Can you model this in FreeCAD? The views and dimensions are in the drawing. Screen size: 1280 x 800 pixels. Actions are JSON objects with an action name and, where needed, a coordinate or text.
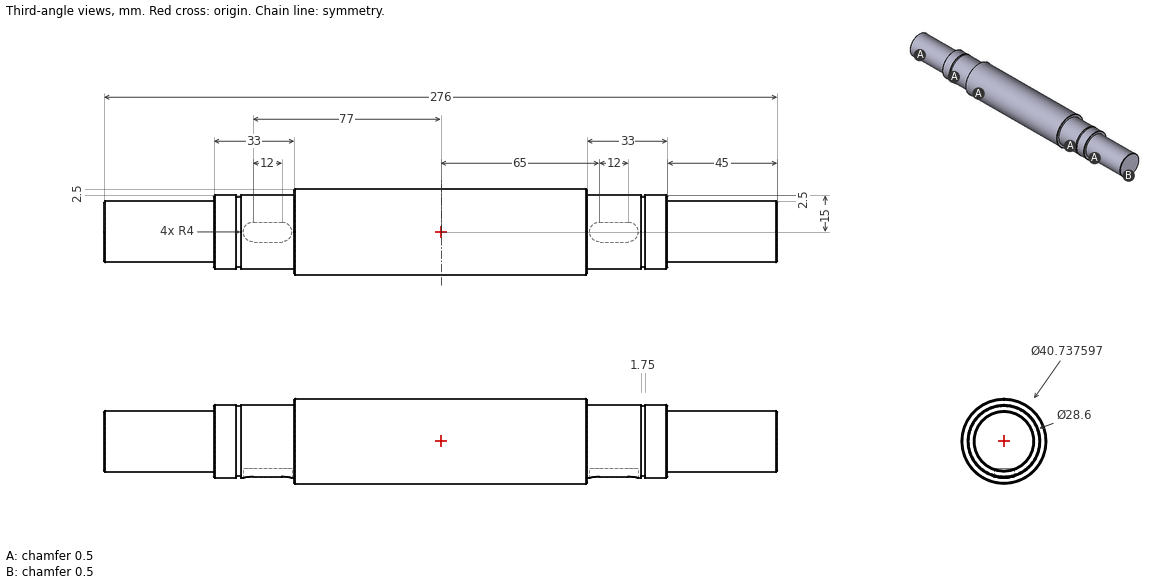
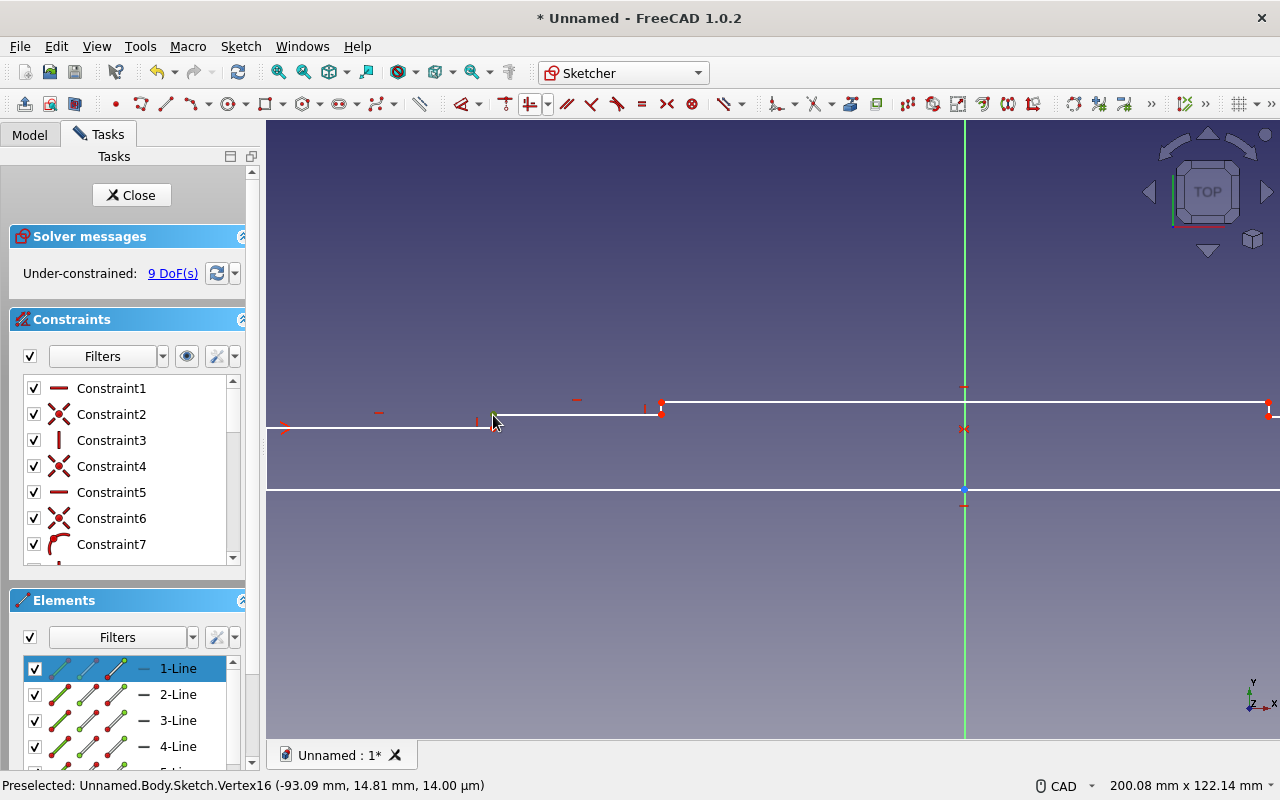
{"action": "left_click", "coordinate": [965, 671]}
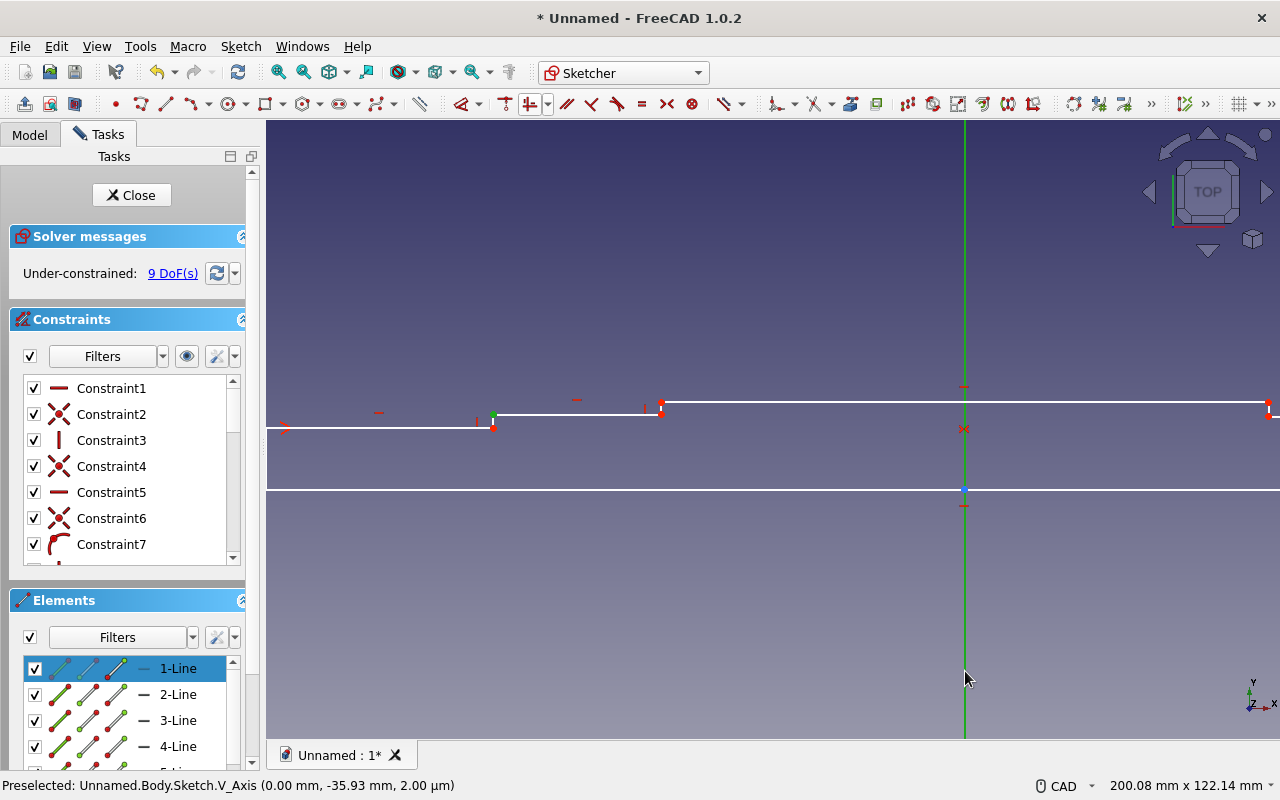
{"action": "left_click", "coordinate": [667, 104]}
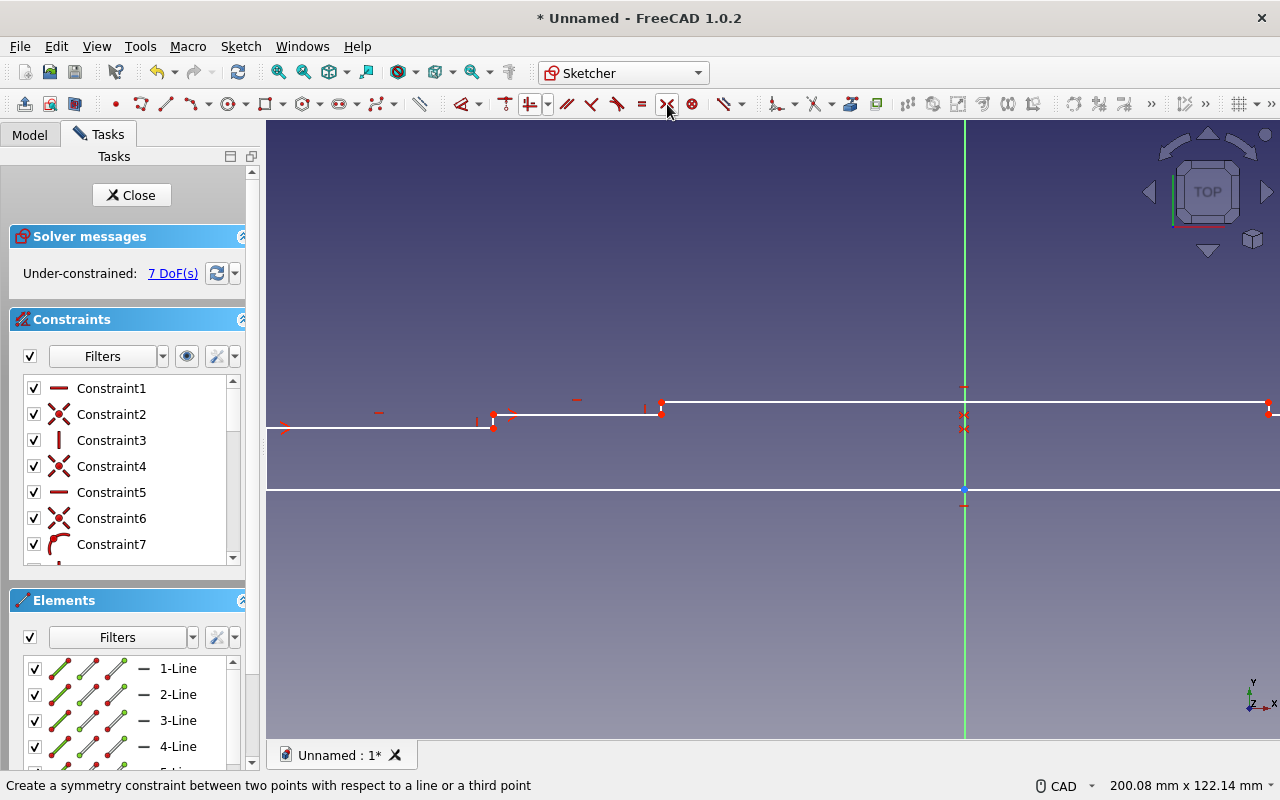
{"action": "left_click", "coordinate": [460, 104]}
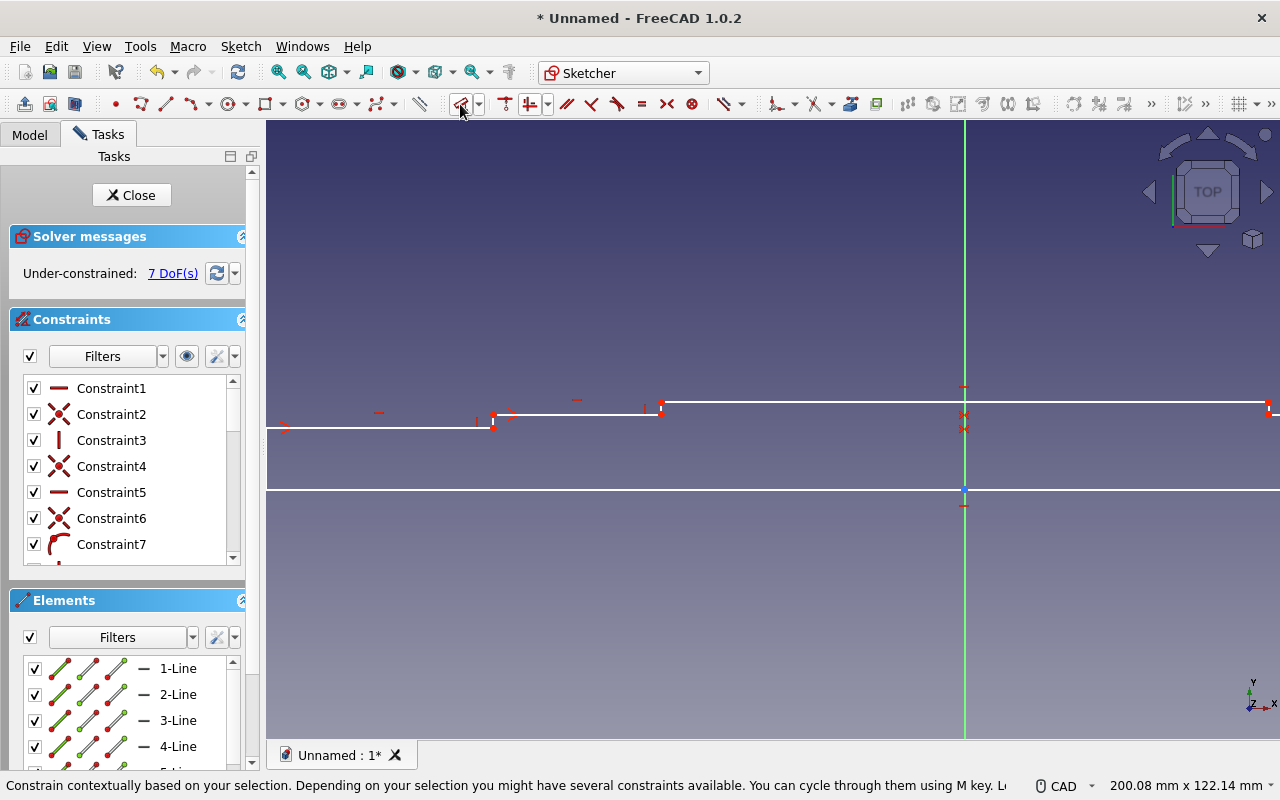
{"action": "scroll", "coordinate": [492, 416], "scroll_direction": "down", "scroll_amount": 4}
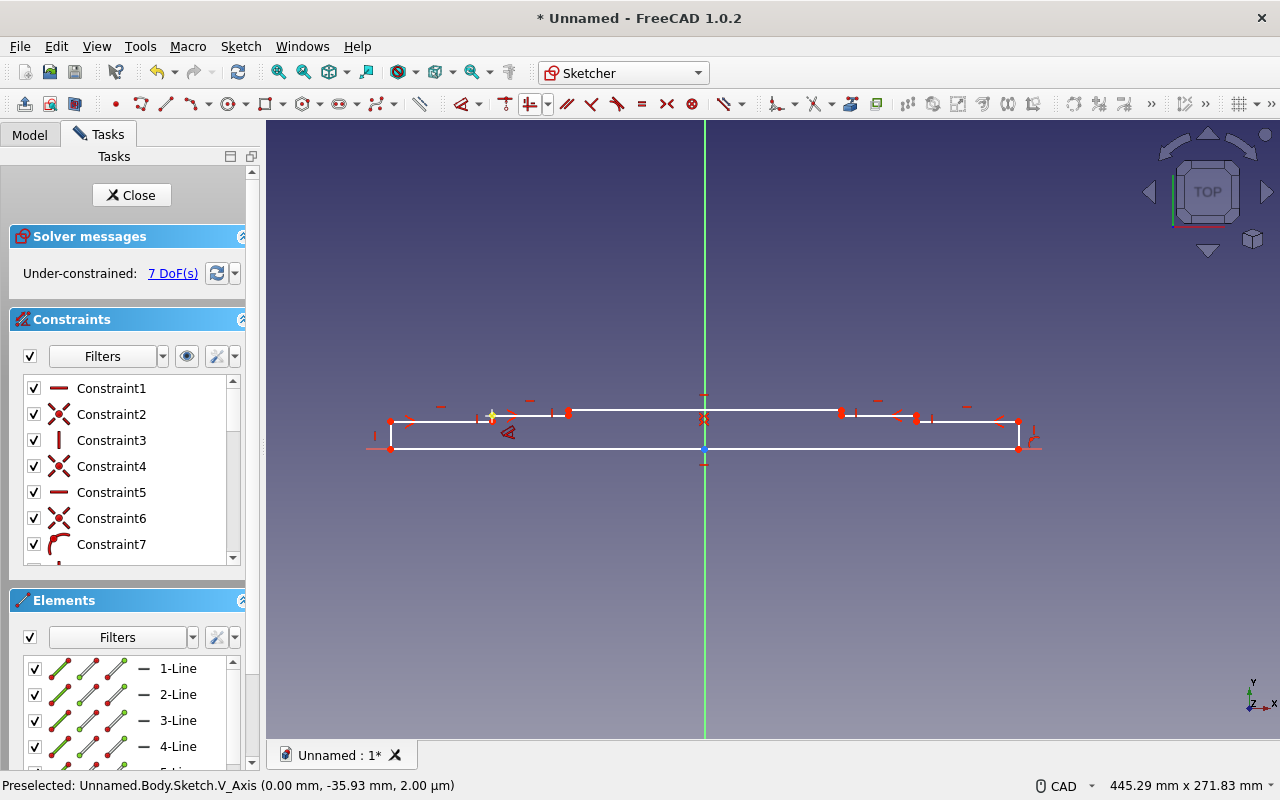
{"action": "left_click", "coordinate": [864, 416]}
{"action": "left_click", "coordinate": [879, 382]}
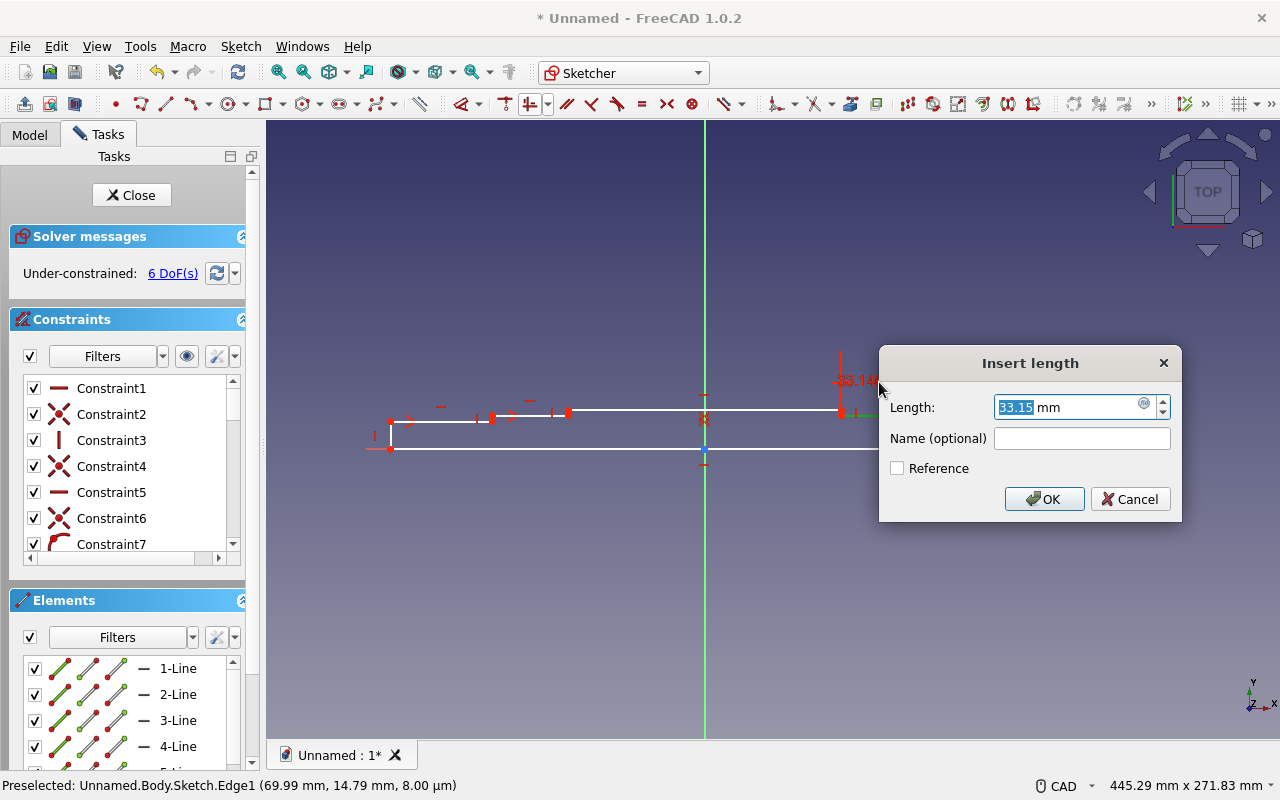
{"action": "type", "text": "33"}
{"action": "key", "text": "Return"}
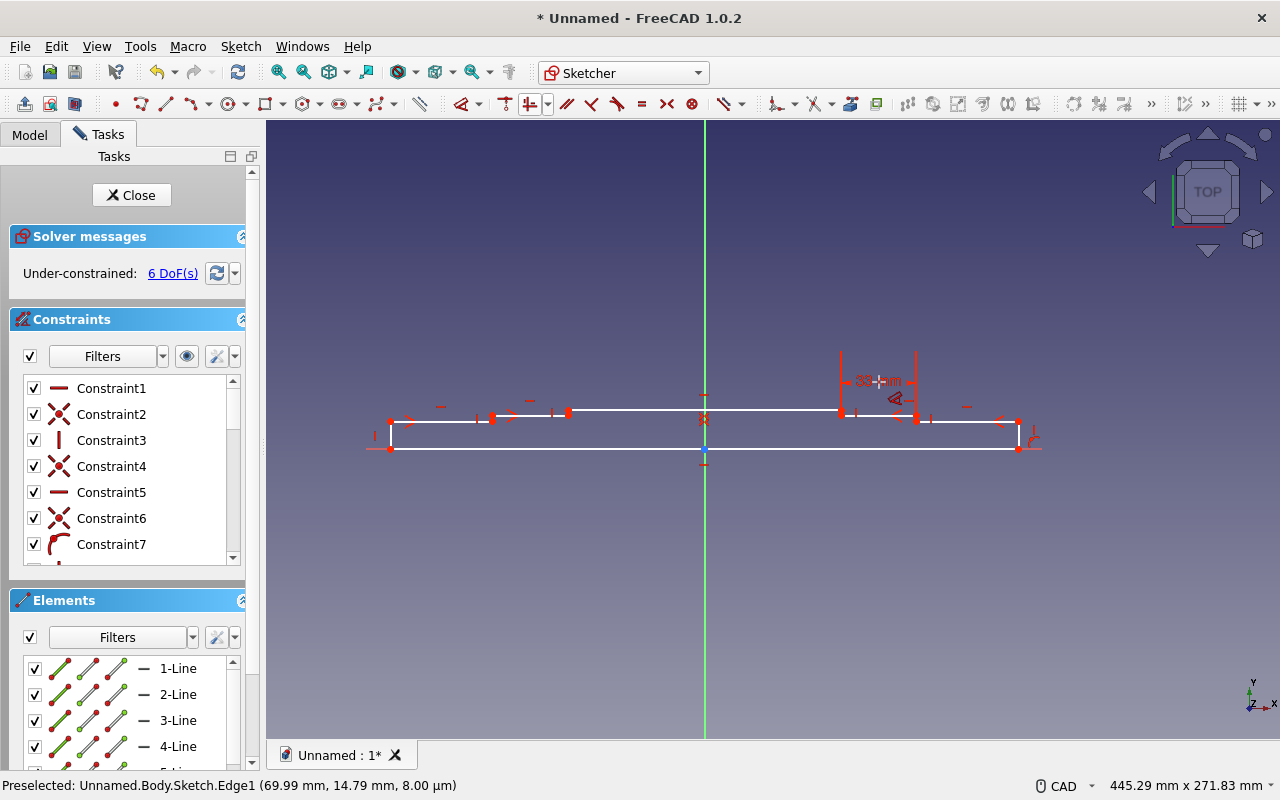
{"action": "left_click", "coordinate": [947, 422]}
{"action": "left_click", "coordinate": [968, 388]}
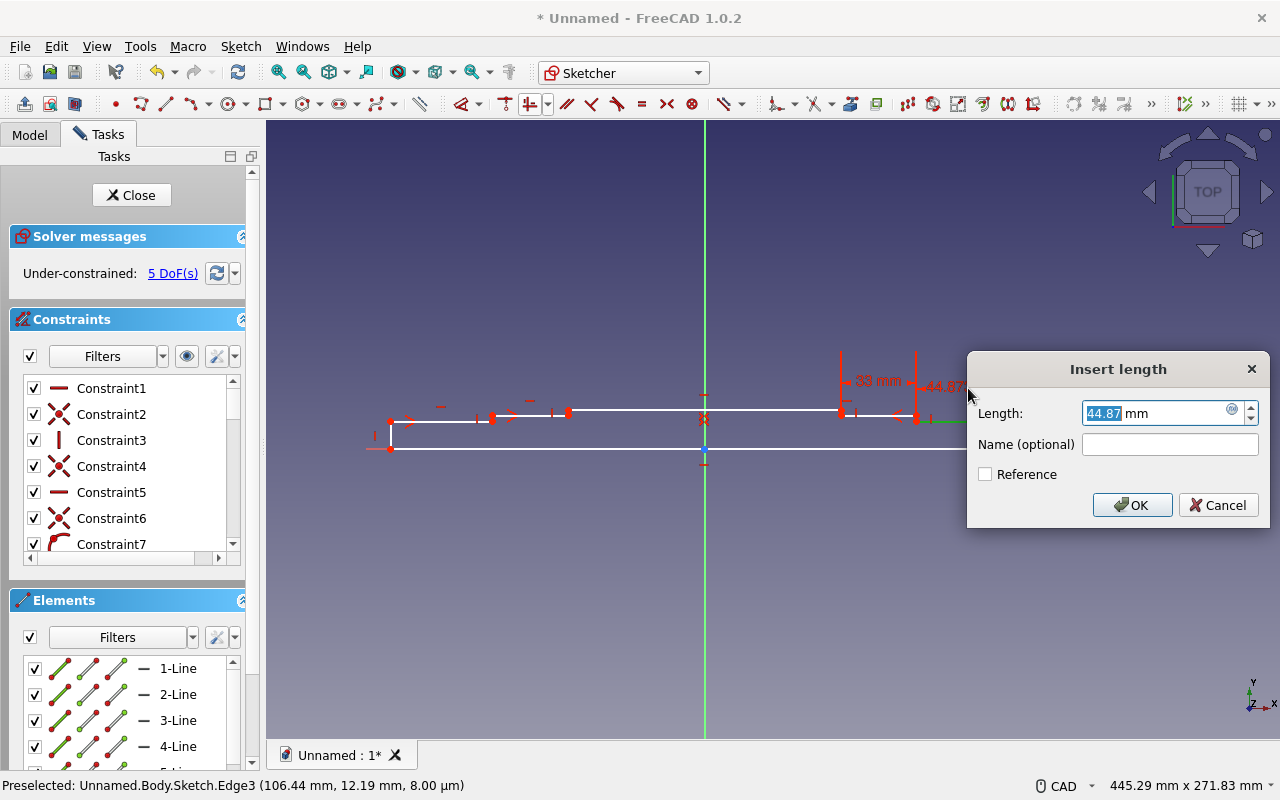
{"action": "type", "text": "45"}
{"action": "key", "text": "Return"}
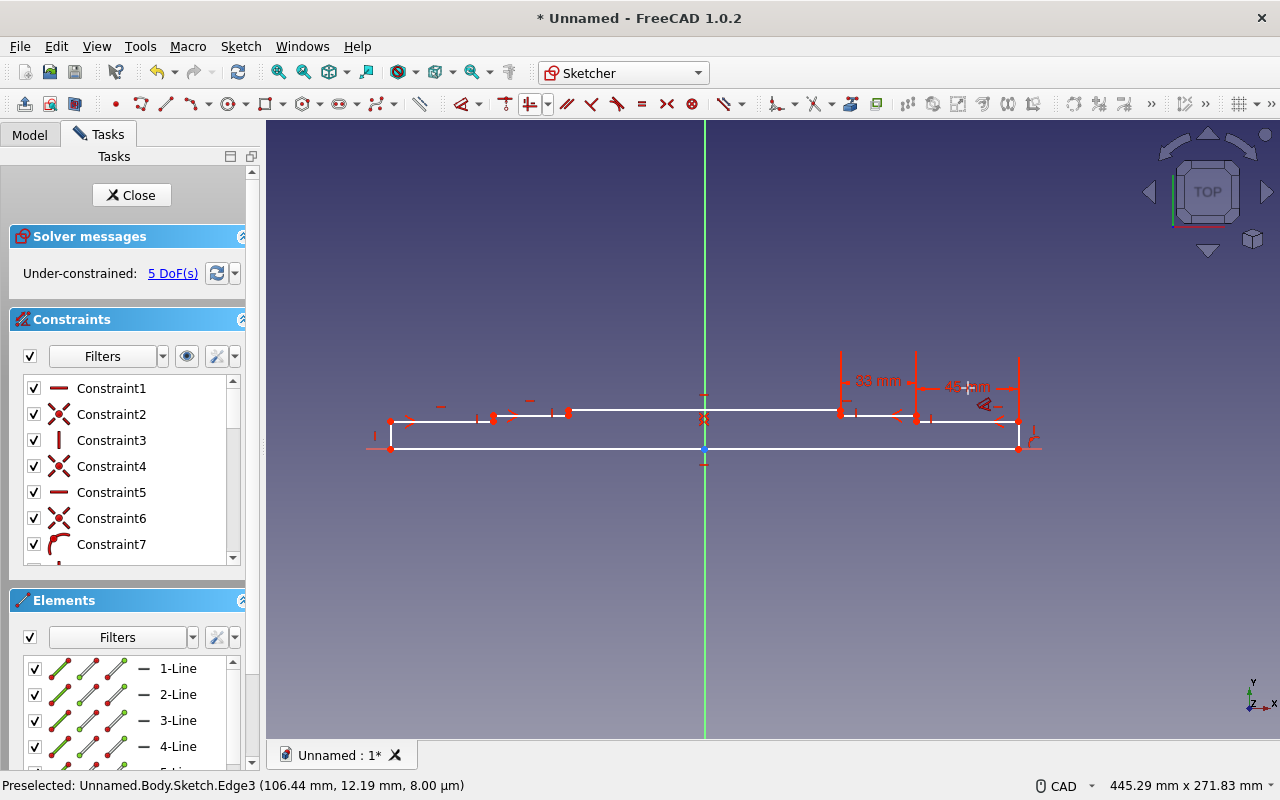
{"action": "left_click", "coordinate": [516, 416]}
{"action": "left_click", "coordinate": [531, 382]}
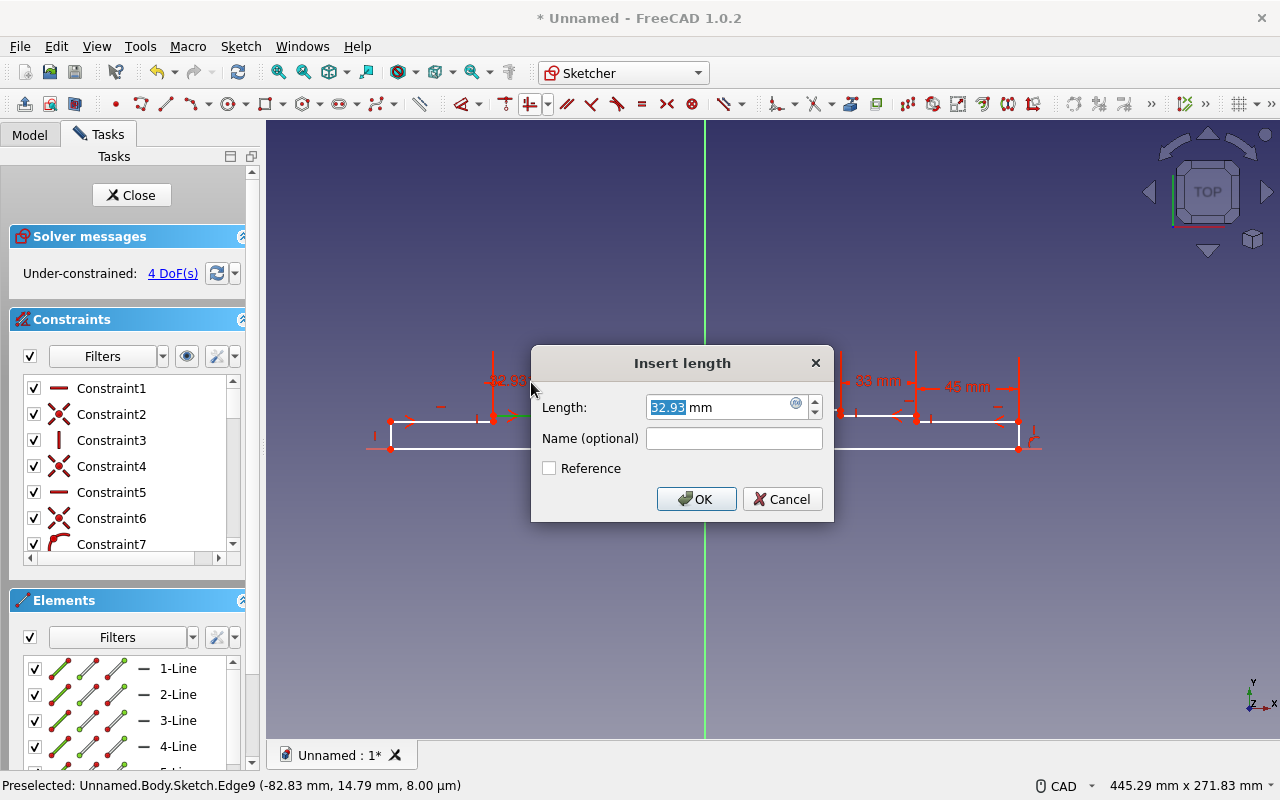
{"action": "type", "text": "33"}
{"action": "key", "text": "Return"}